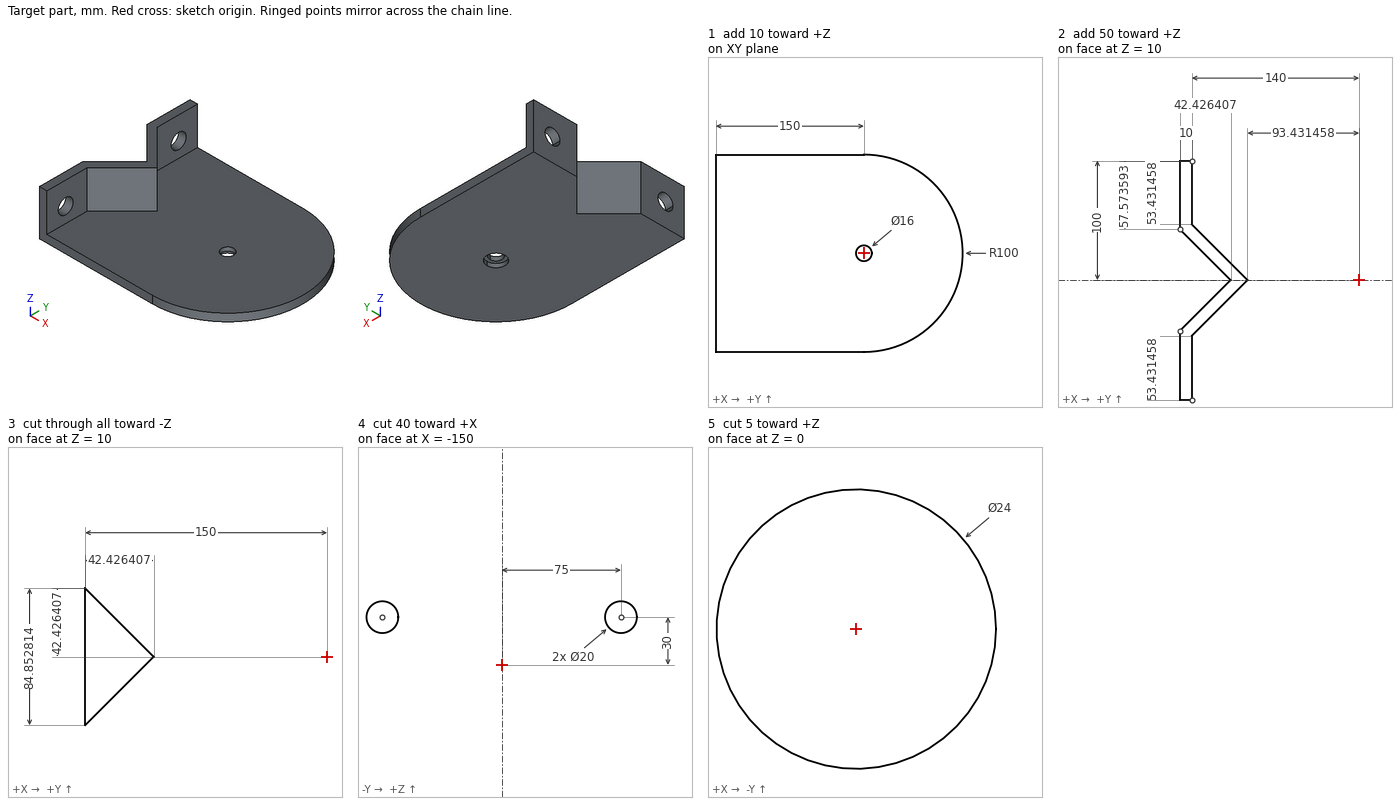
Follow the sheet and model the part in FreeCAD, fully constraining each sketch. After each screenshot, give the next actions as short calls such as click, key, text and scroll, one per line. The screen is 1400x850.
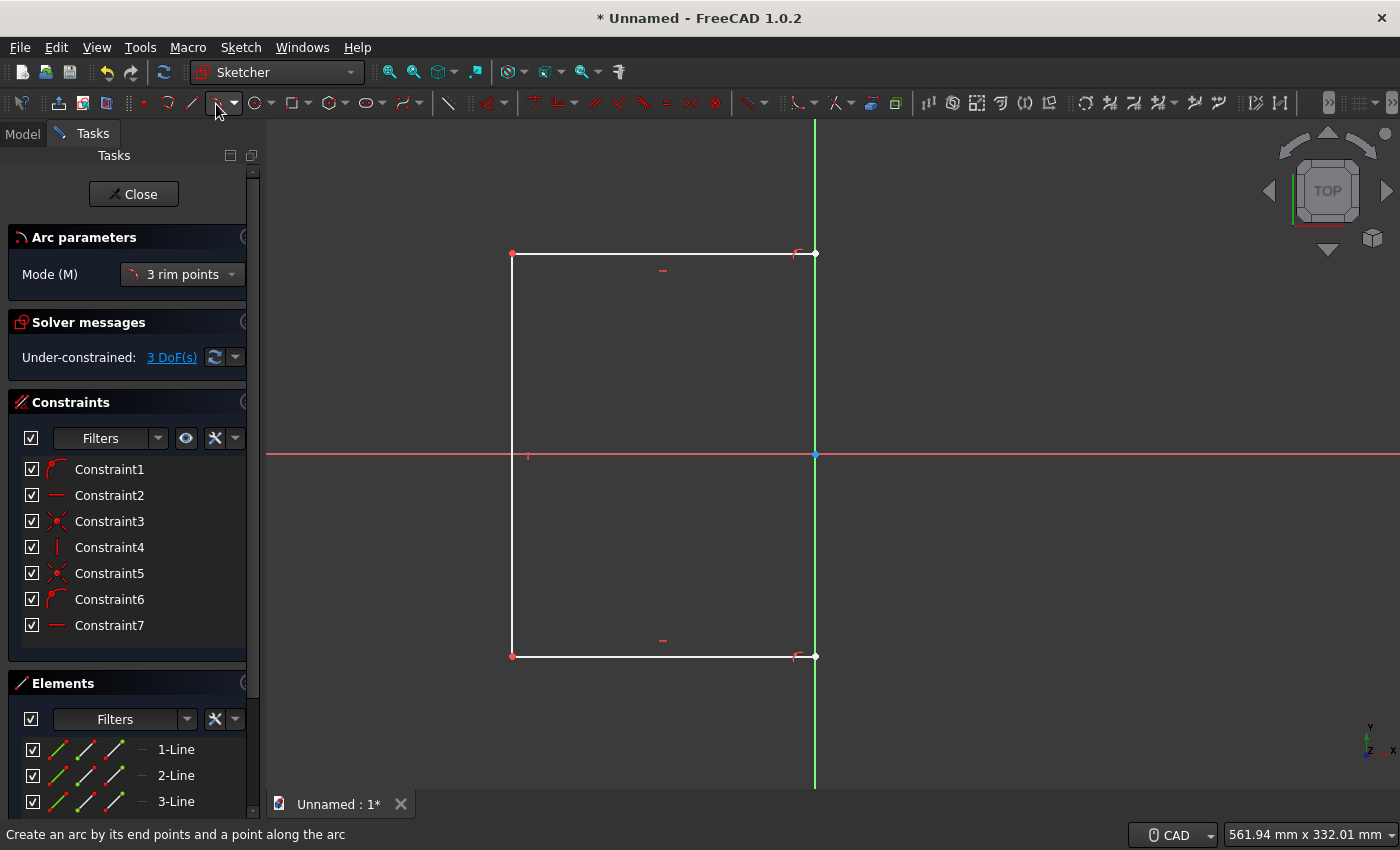
click(815, 657)
click(815, 254)
click(1007, 517)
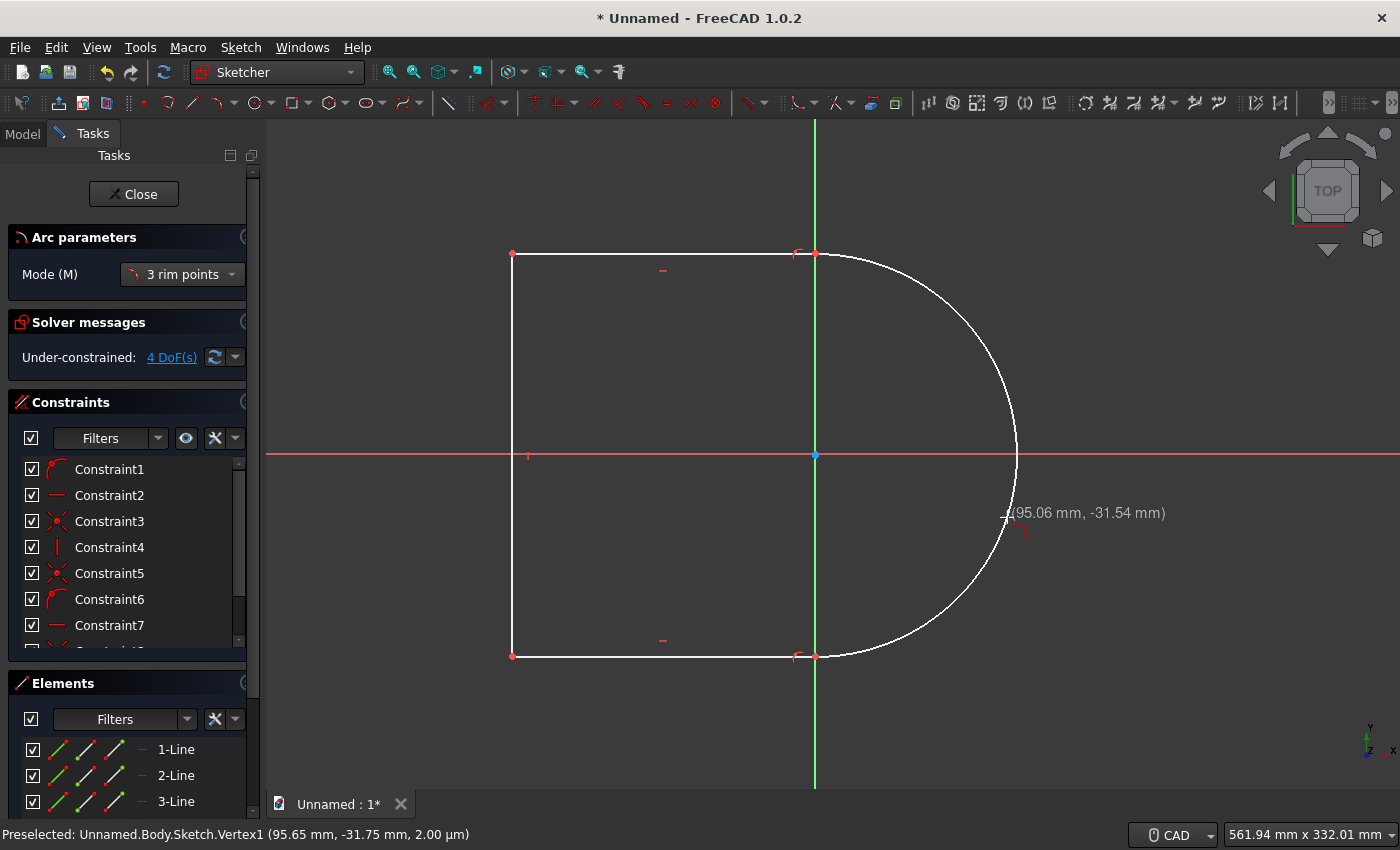
key(g)
key(c)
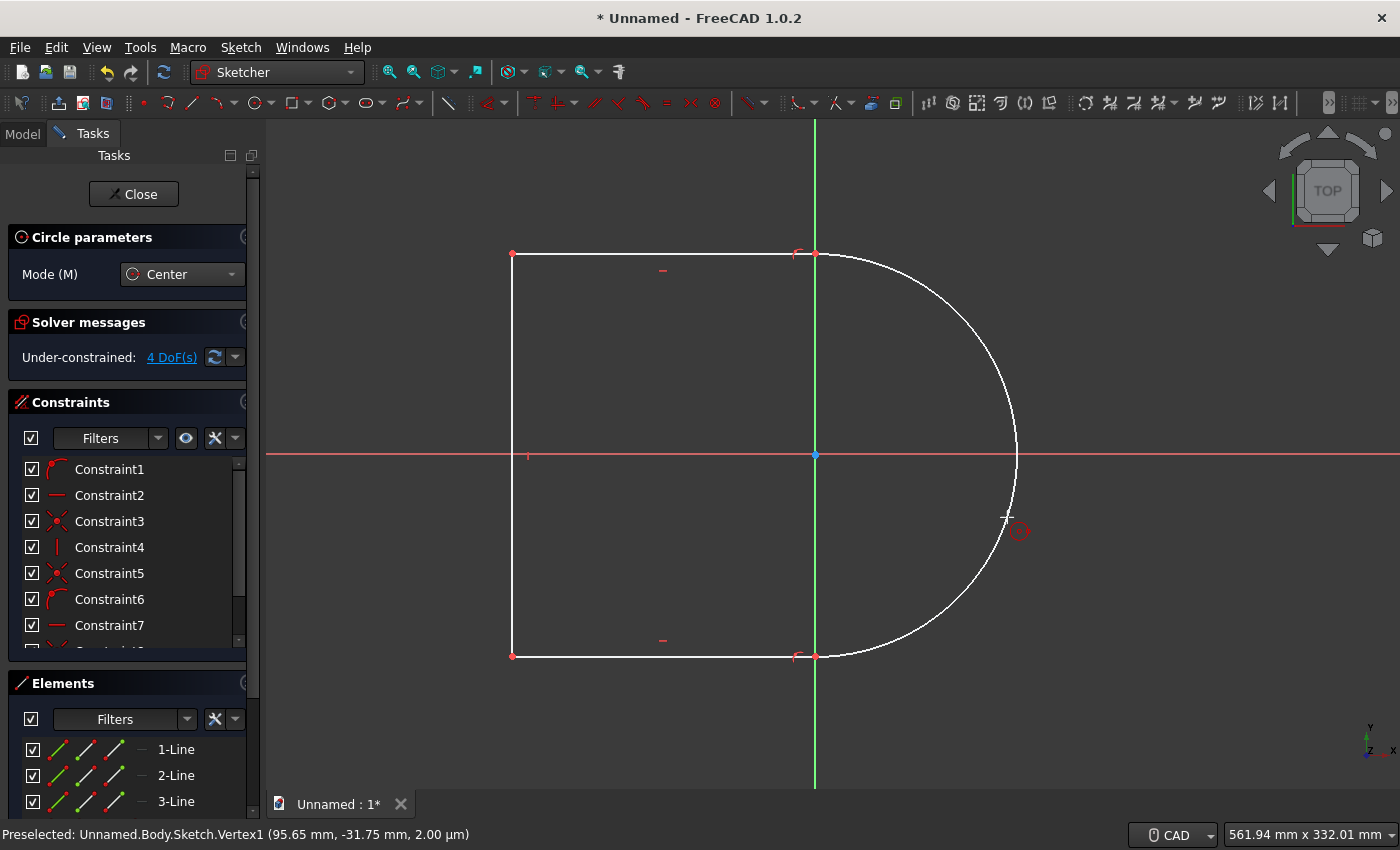
scroll(815, 454, up, 2)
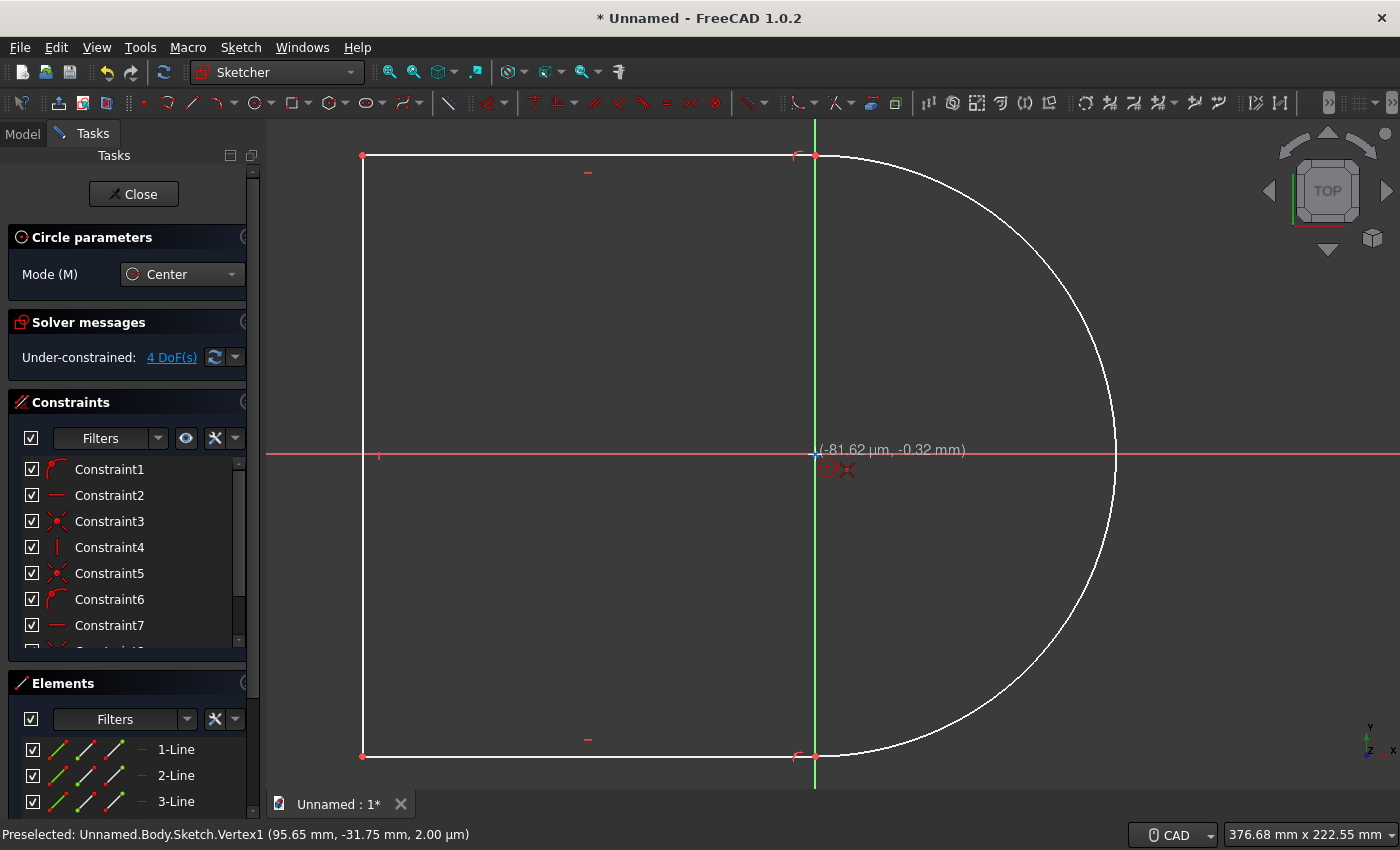
click(815, 454)
click(832, 437)
key(Escape)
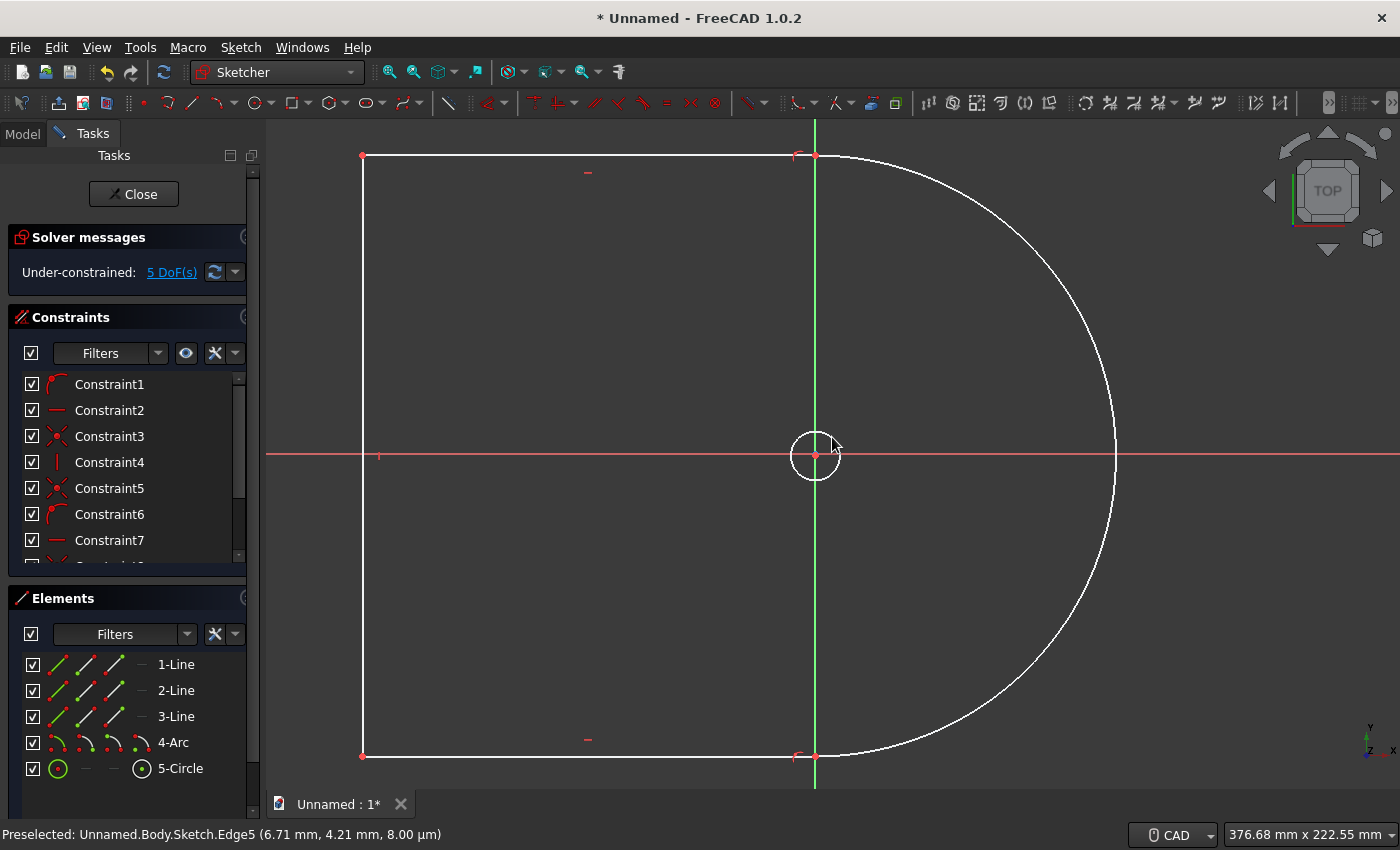
scroll(815, 455, up, 3)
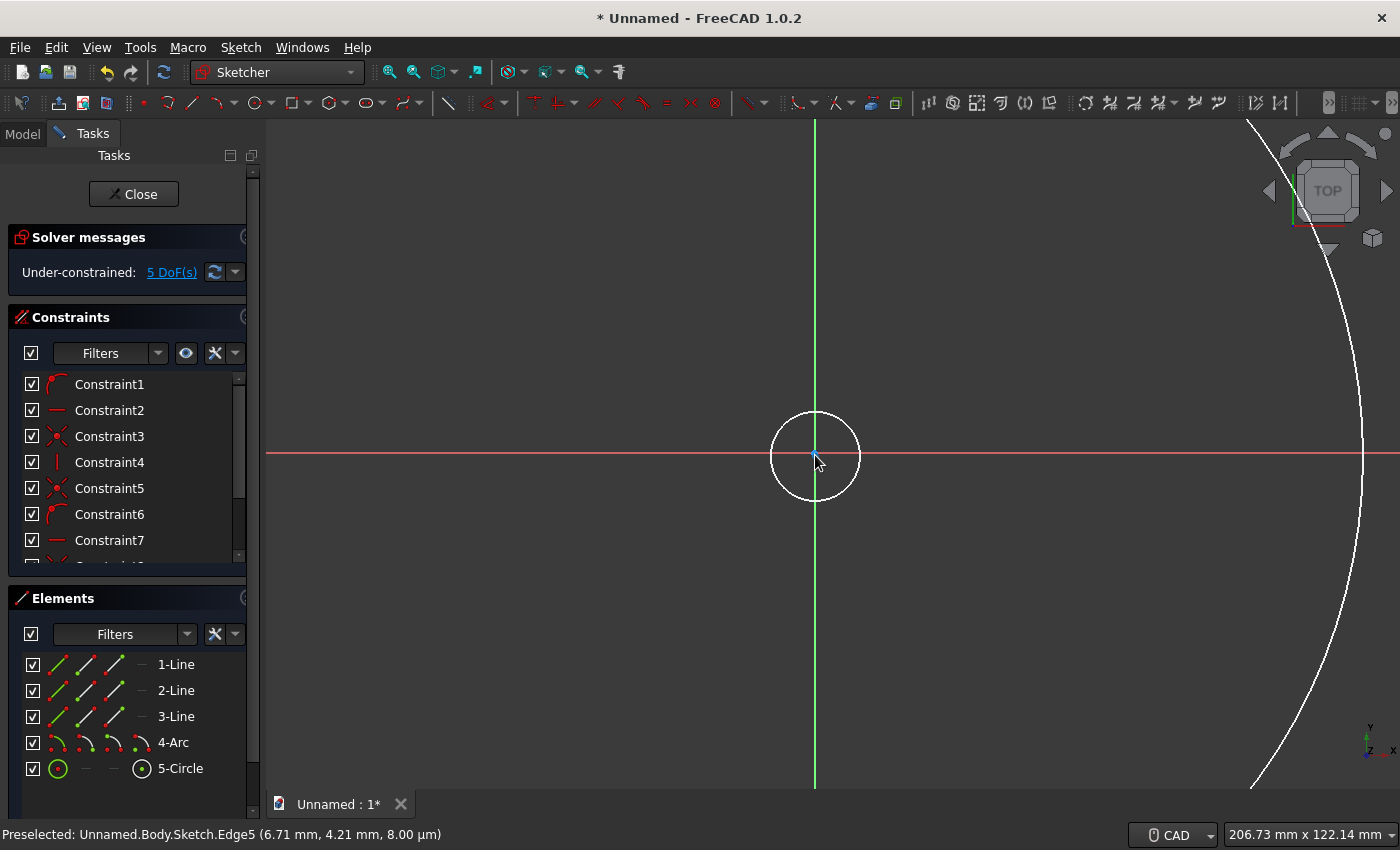
drag(805, 443, 825, 466)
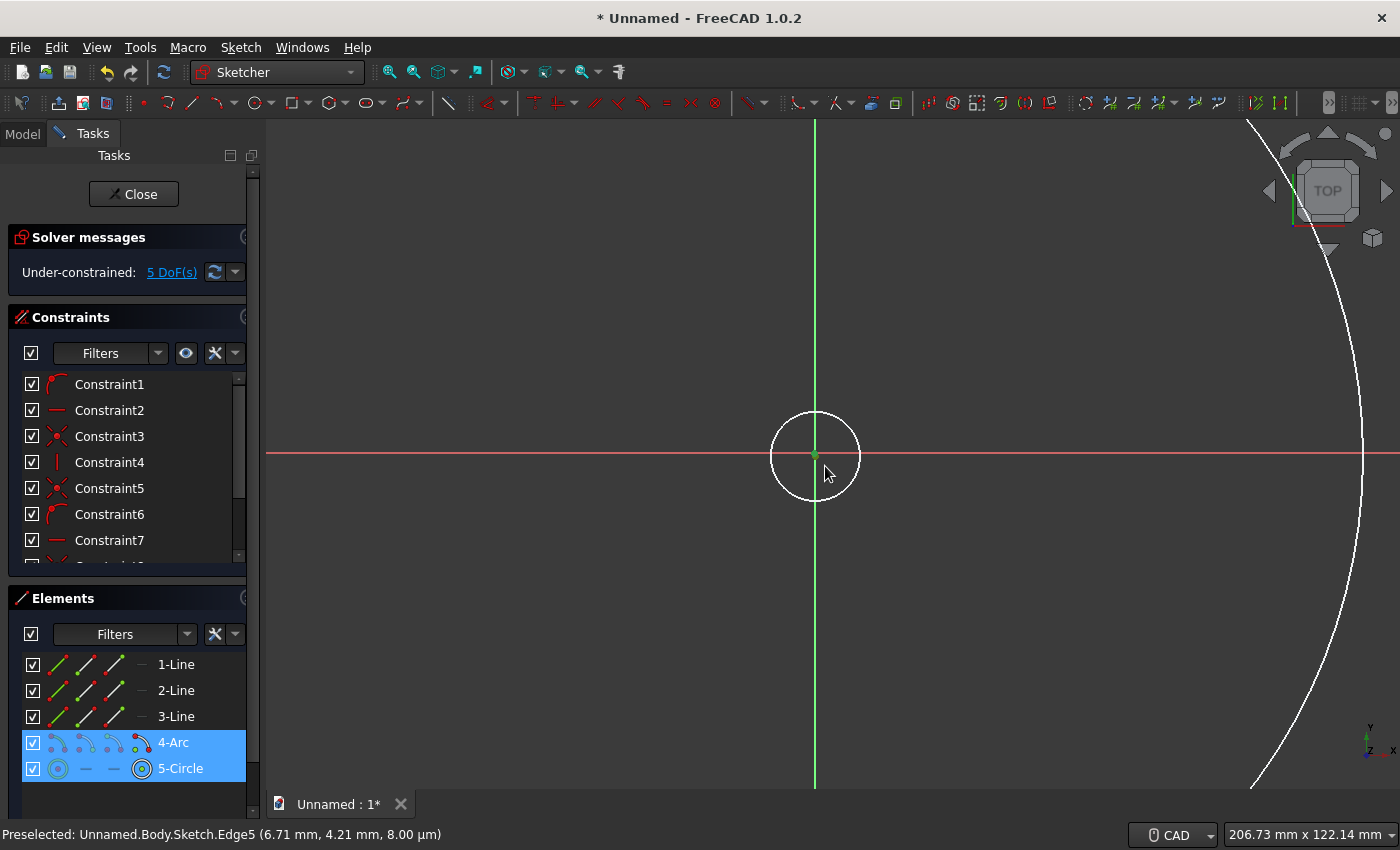
key(c)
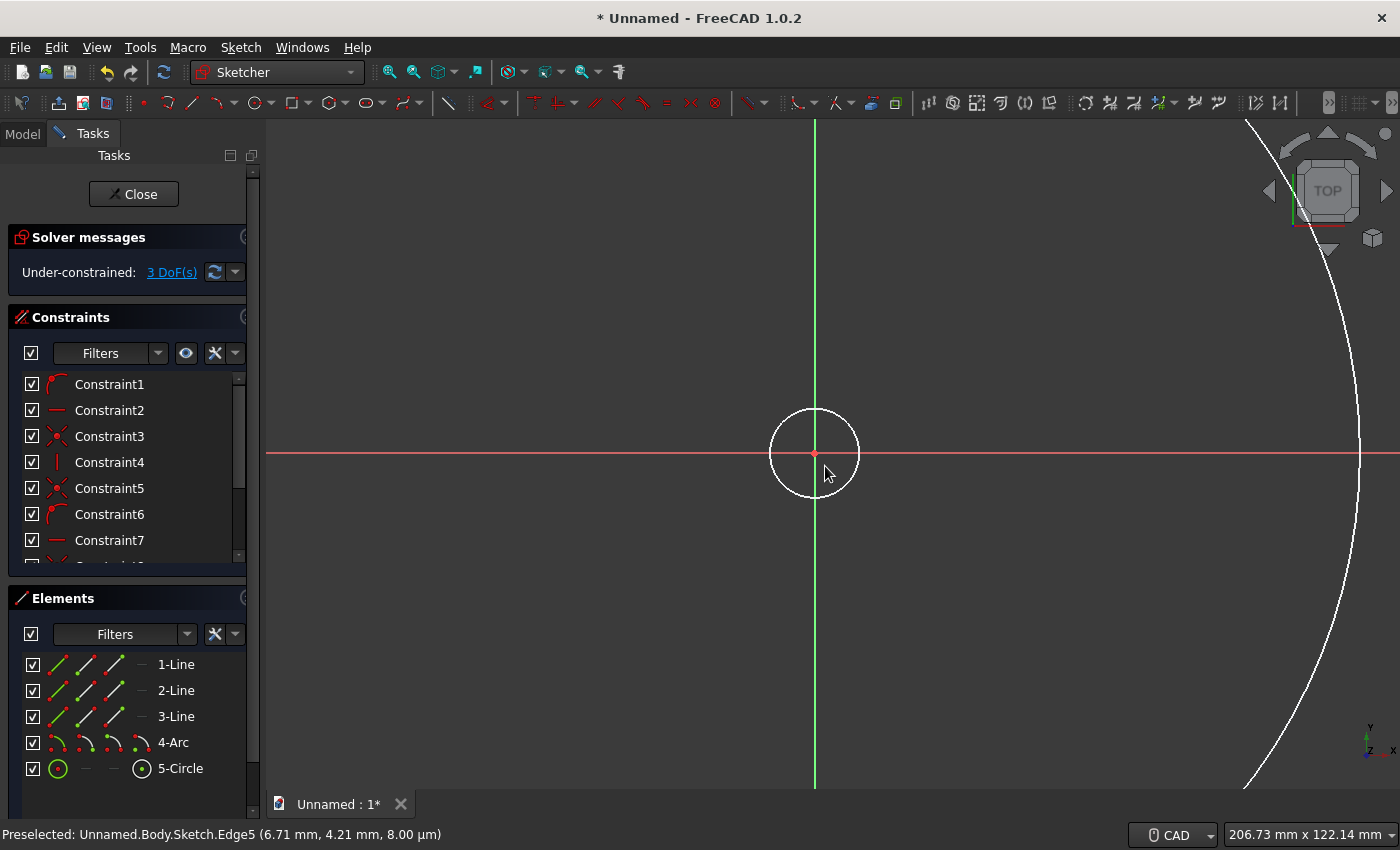
key(d)